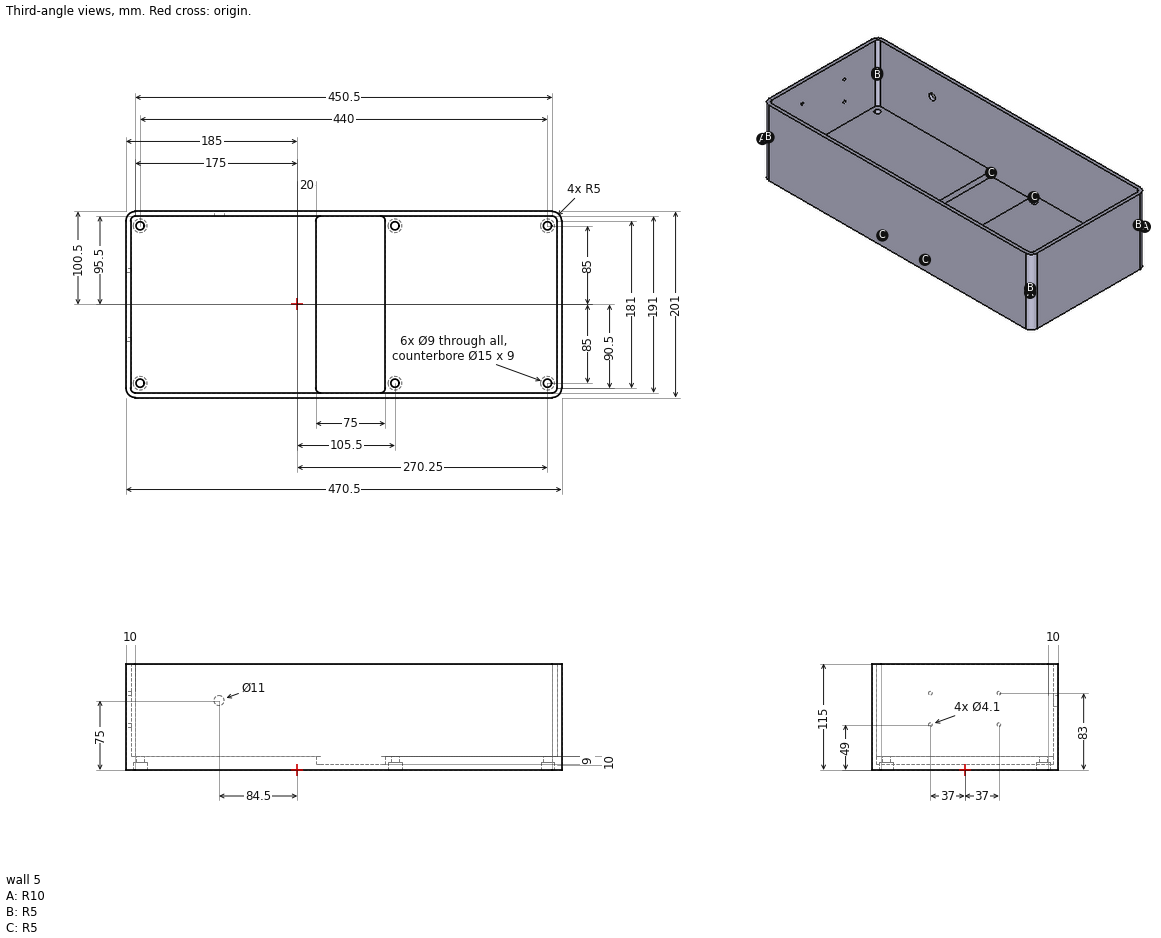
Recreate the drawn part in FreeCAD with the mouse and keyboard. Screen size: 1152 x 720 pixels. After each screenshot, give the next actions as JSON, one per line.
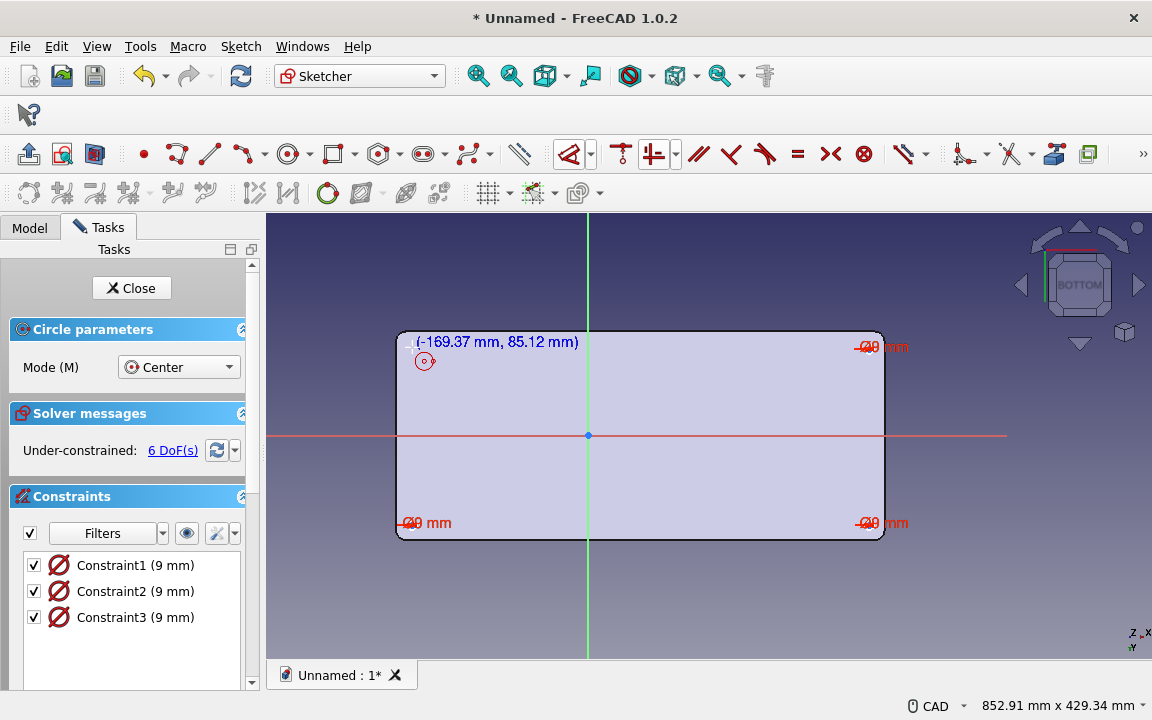
{"action": "left_click", "coordinate": [412, 348]}
{"action": "mouse_move", "coordinate": [415, 344]}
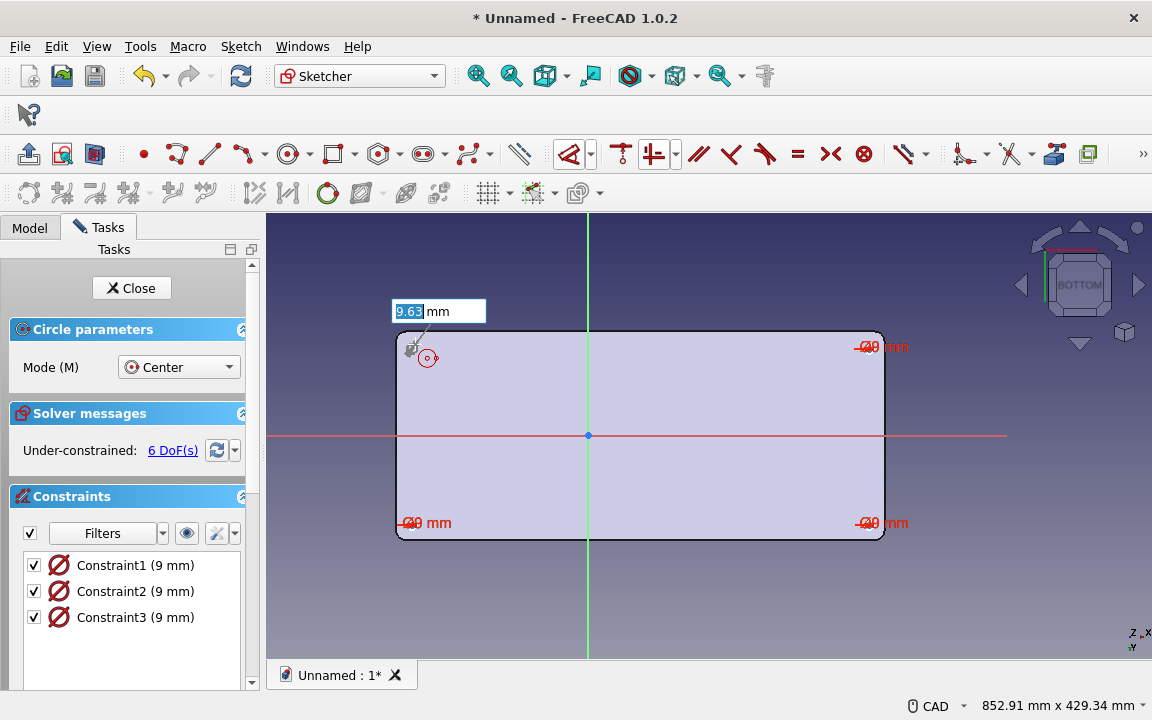
{"action": "type", "text": "9"}
{"action": "key", "text": "Return"}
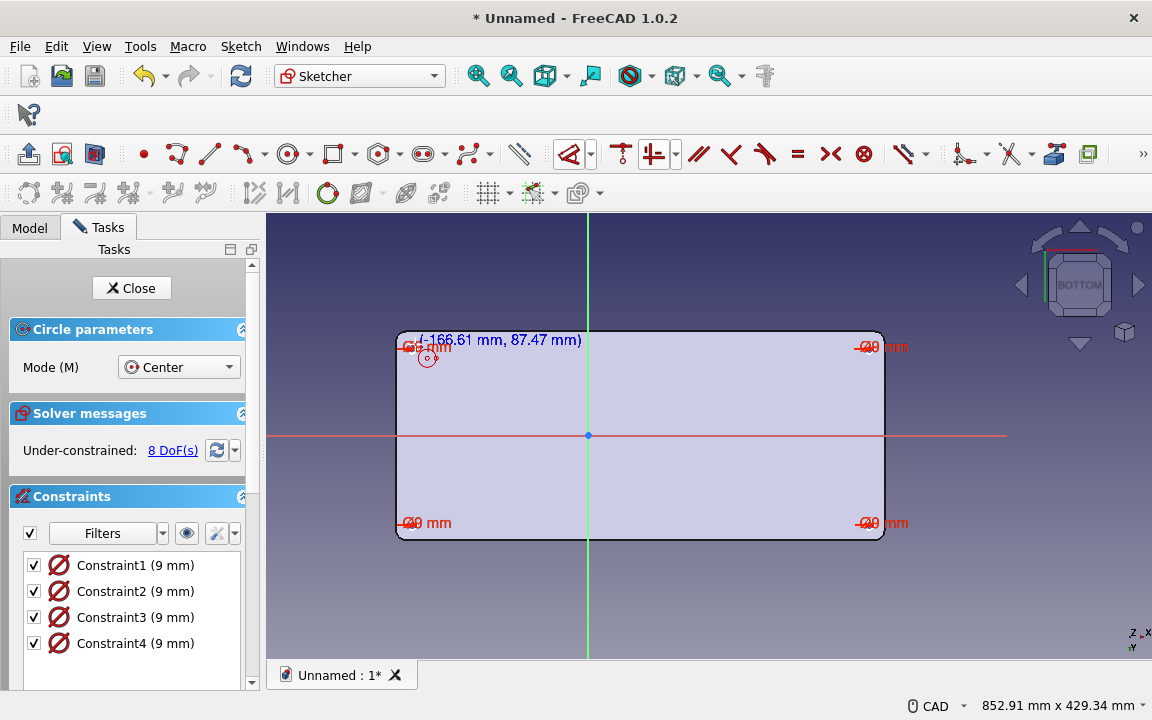
{"action": "scroll", "coordinate": [698, 348], "scroll_direction": "up", "scroll_amount": 8}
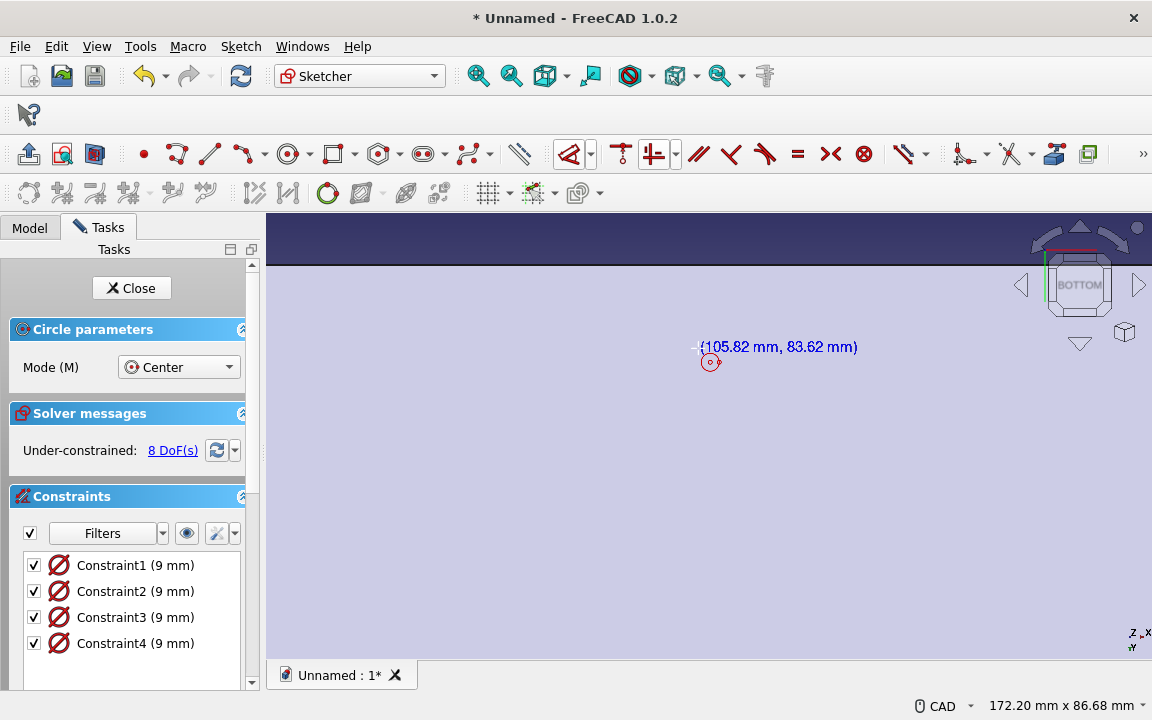
{"action": "scroll", "coordinate": [699, 348], "scroll_direction": "down", "scroll_amount": 8}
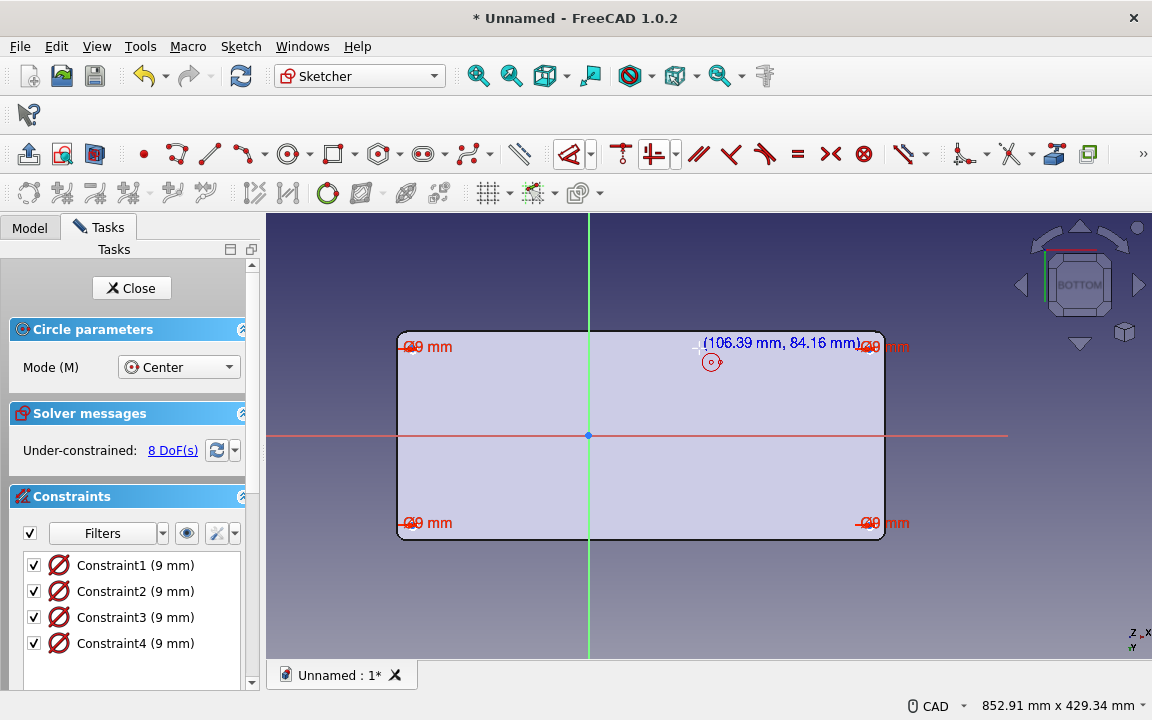
{"action": "left_click", "coordinate": [698, 348]}
{"action": "mouse_move", "coordinate": [702, 344]}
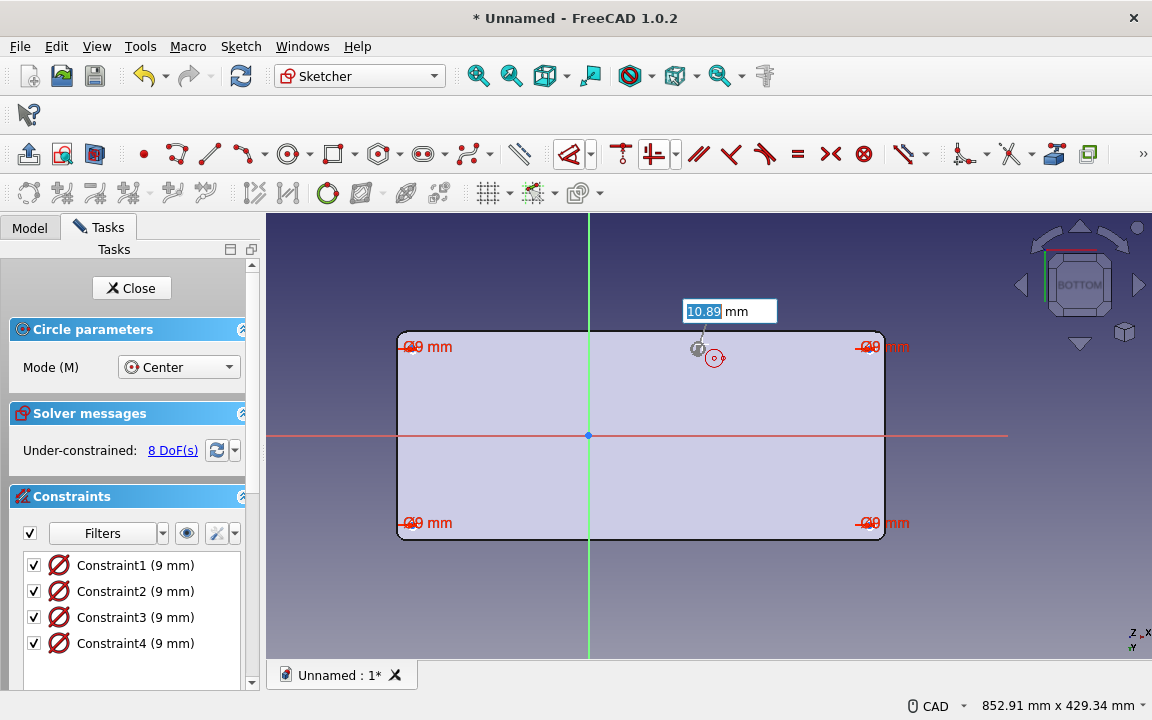
{"action": "type", "text": "9"}
{"action": "key", "text": "Return"}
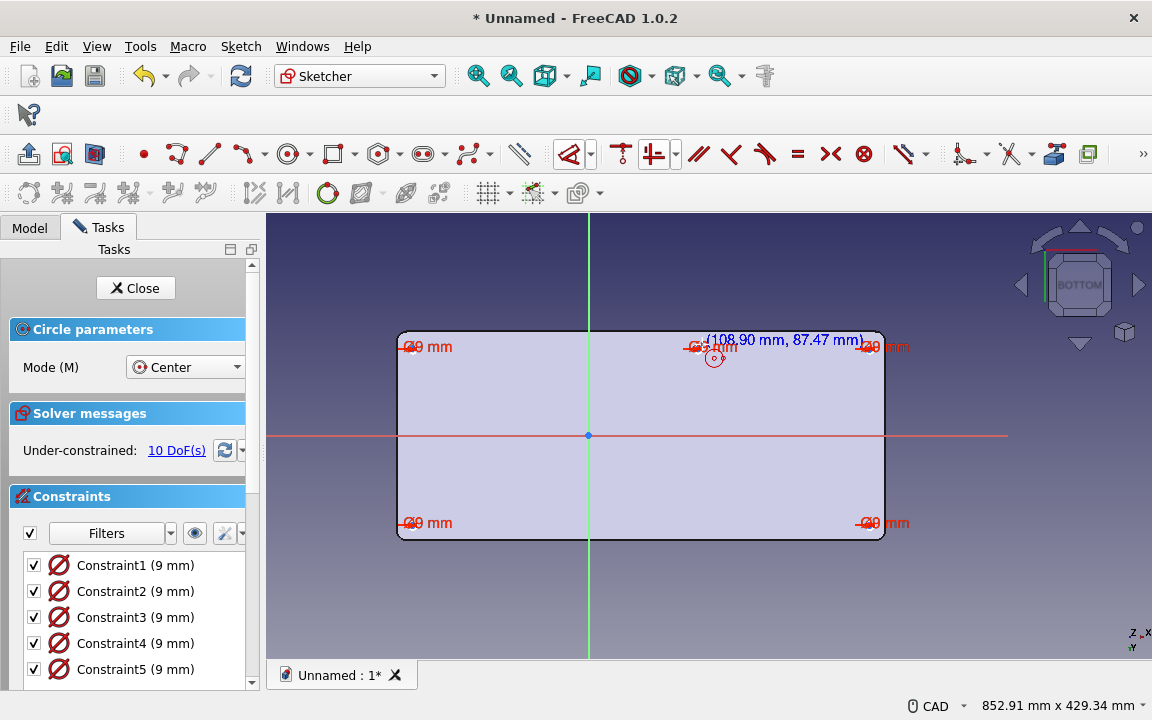
{"action": "scroll", "coordinate": [698, 524], "scroll_direction": "up", "scroll_amount": 8}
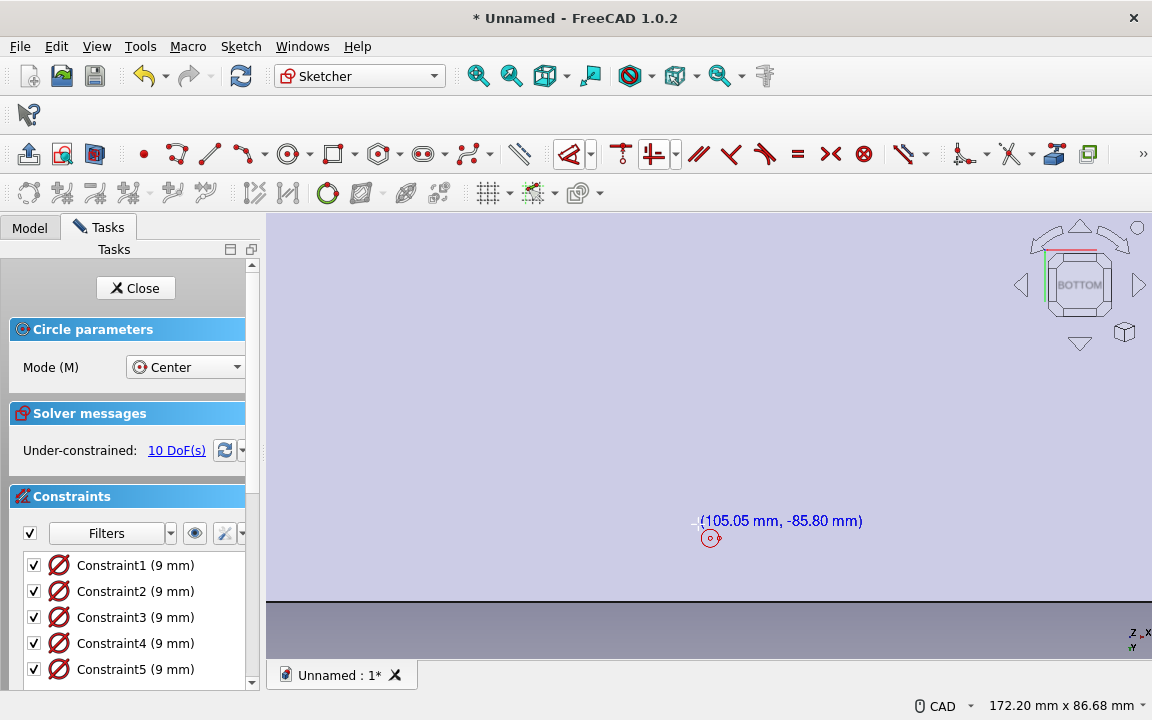
{"action": "scroll", "coordinate": [698, 525], "scroll_direction": "down", "scroll_amount": 8}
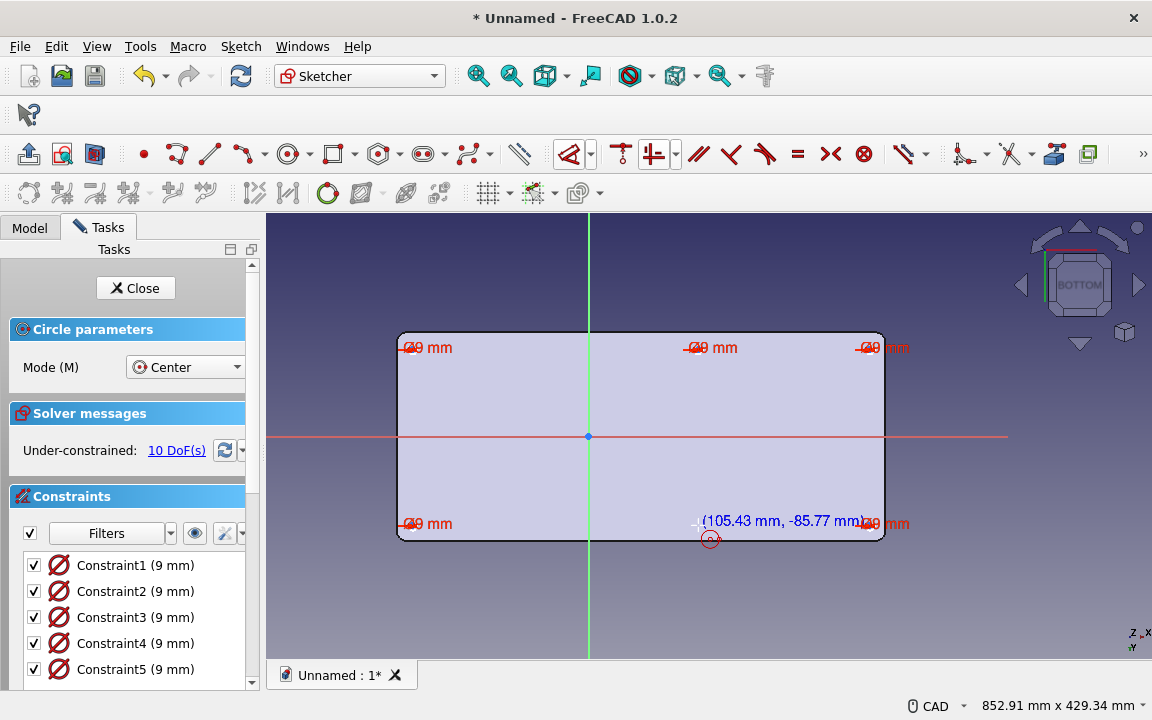
{"action": "left_click", "coordinate": [698, 525]}
{"action": "mouse_move", "coordinate": [702, 522]}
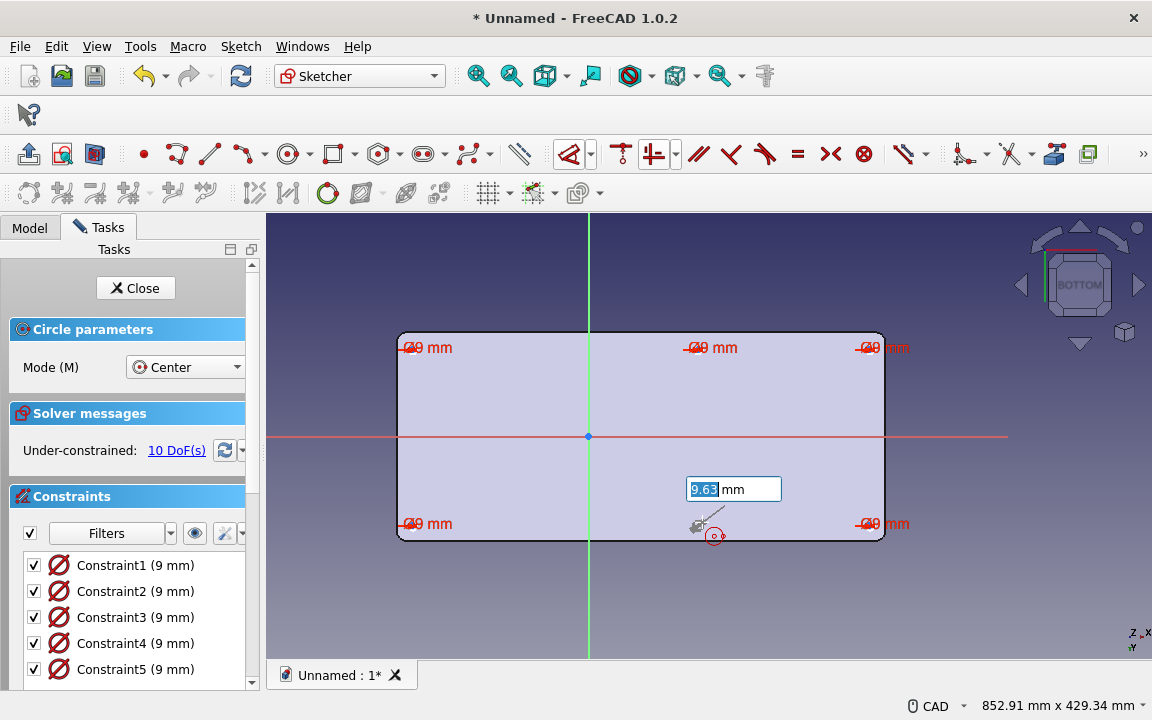
{"action": "type", "text": "9"}
{"action": "key", "text": "Return"}
{"action": "key", "text": "Escape"}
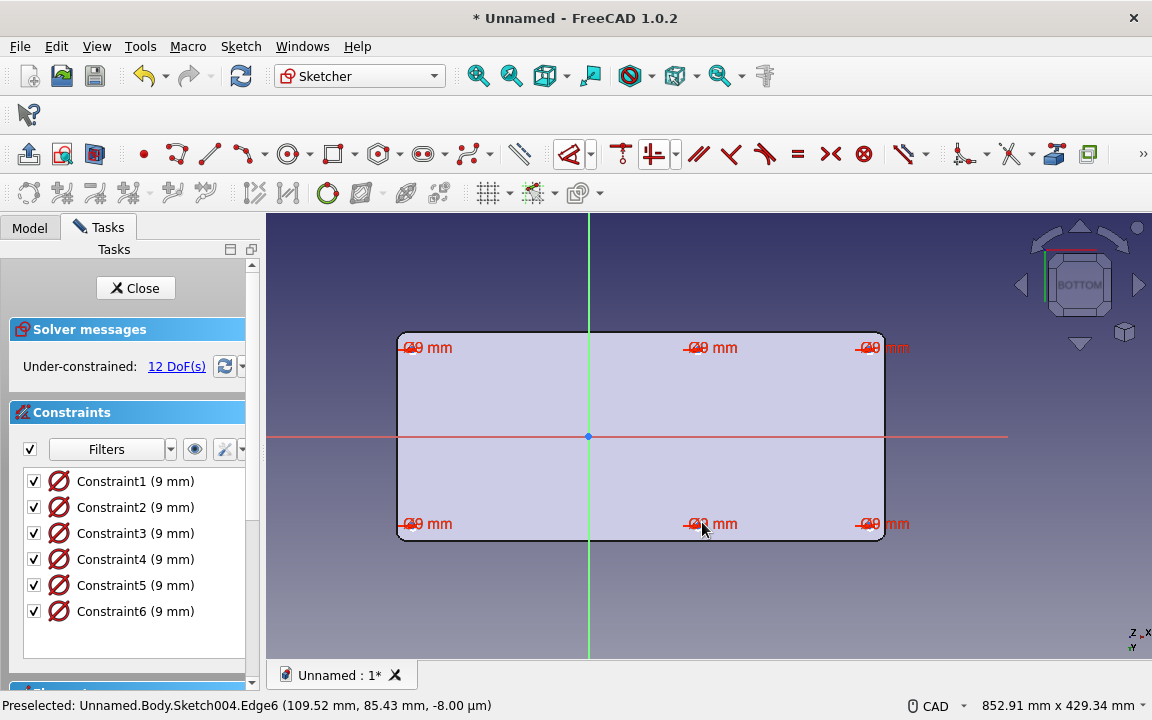
{"action": "left_click", "coordinate": [870, 350]}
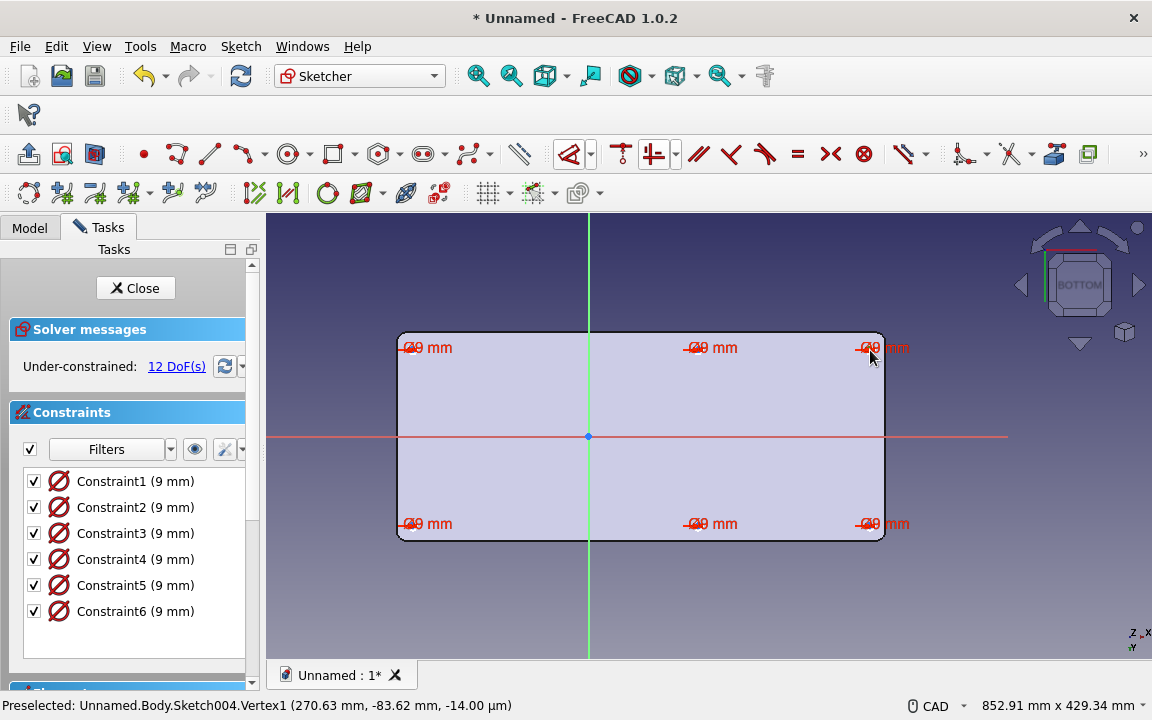
{"action": "left_click", "coordinate": [870, 526]}